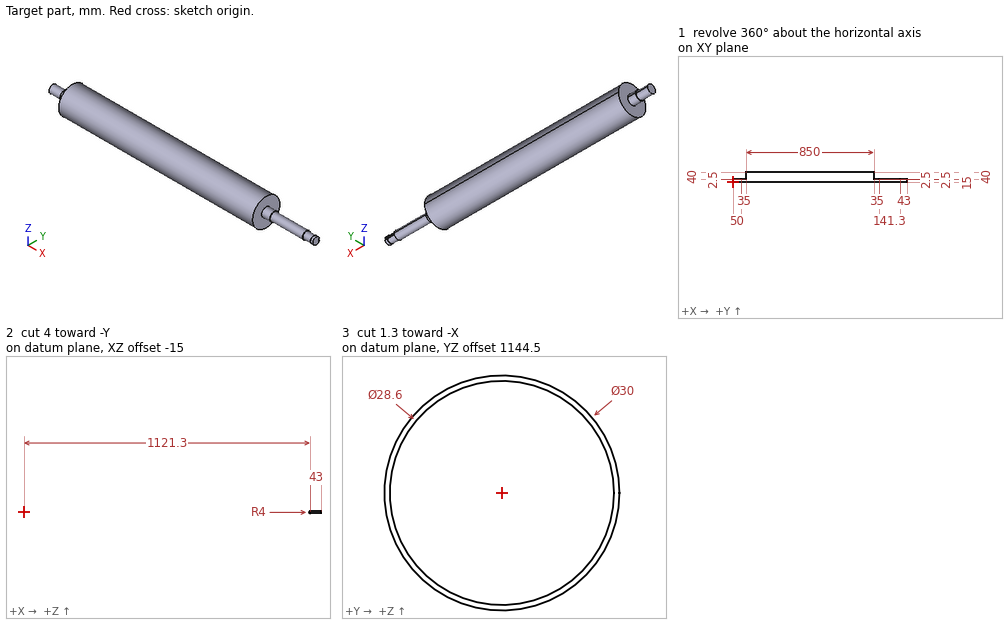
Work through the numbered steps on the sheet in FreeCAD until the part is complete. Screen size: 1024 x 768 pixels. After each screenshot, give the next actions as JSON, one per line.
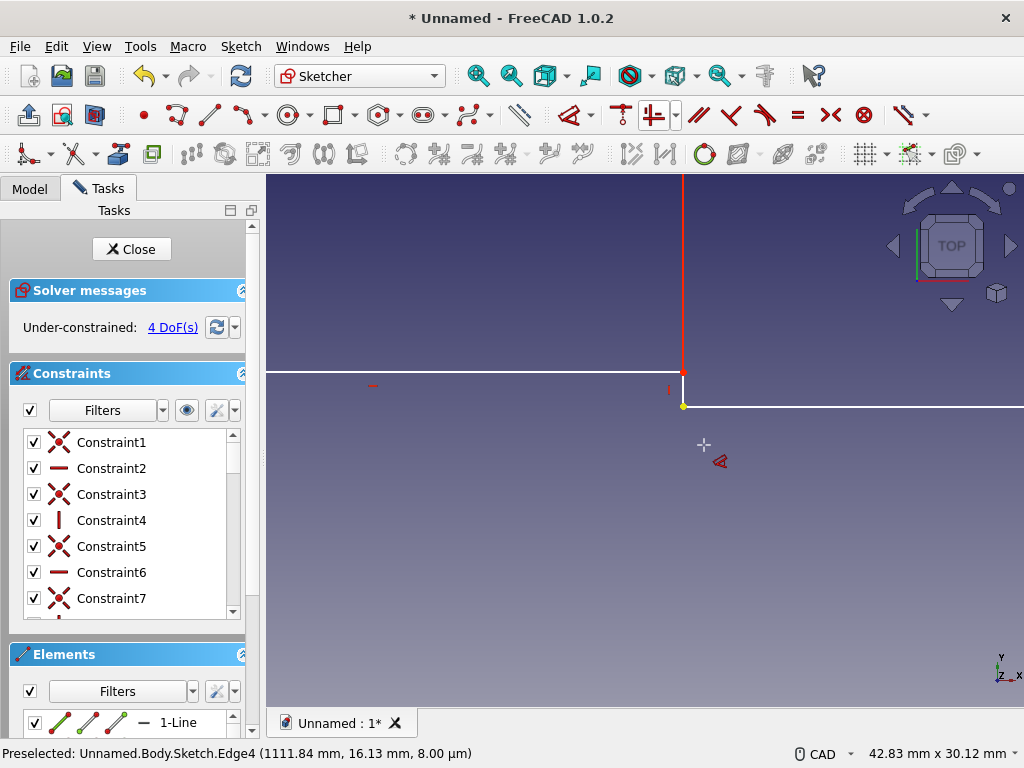
{"action": "left_click", "coordinate": [683, 396]}
{"action": "left_click", "coordinate": [717, 389]}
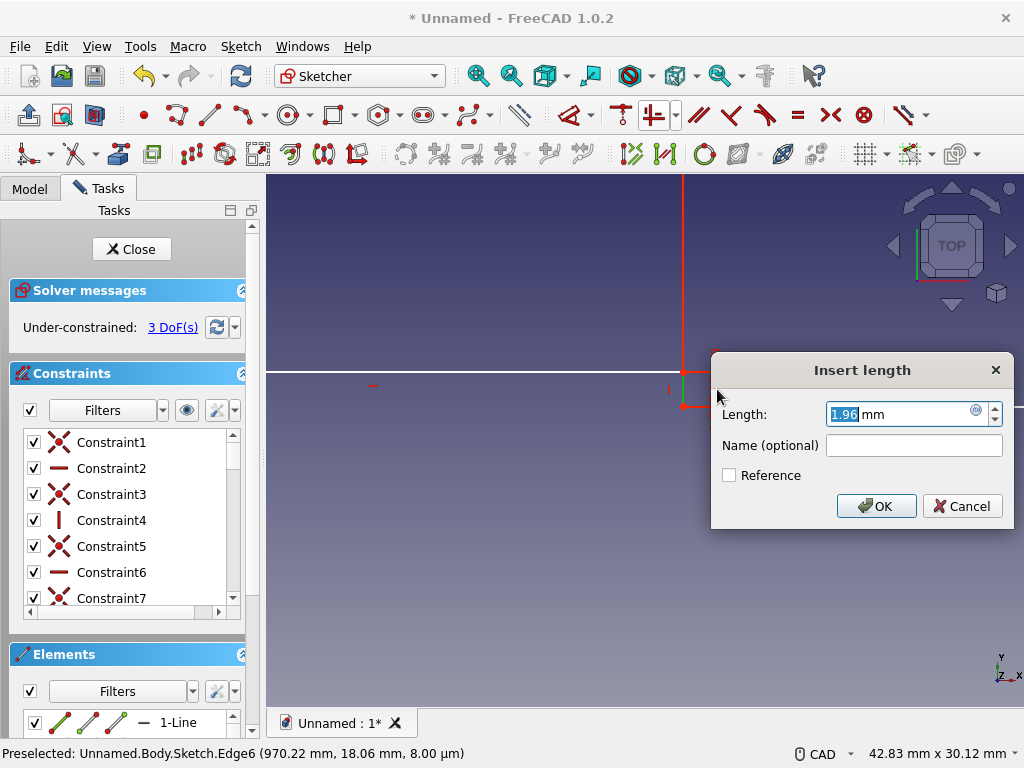
{"action": "type", "text": "2.5"}
{"action": "key", "text": "Return"}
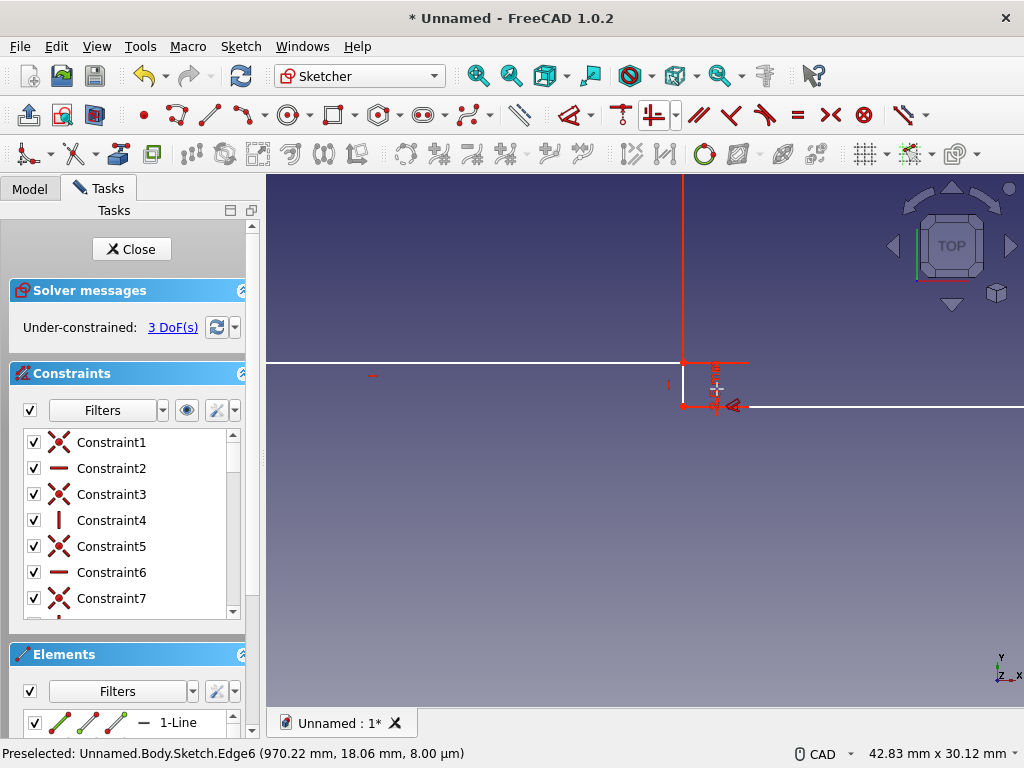
{"action": "scroll", "coordinate": [576, 440], "scroll_direction": "down", "scroll_amount": 15}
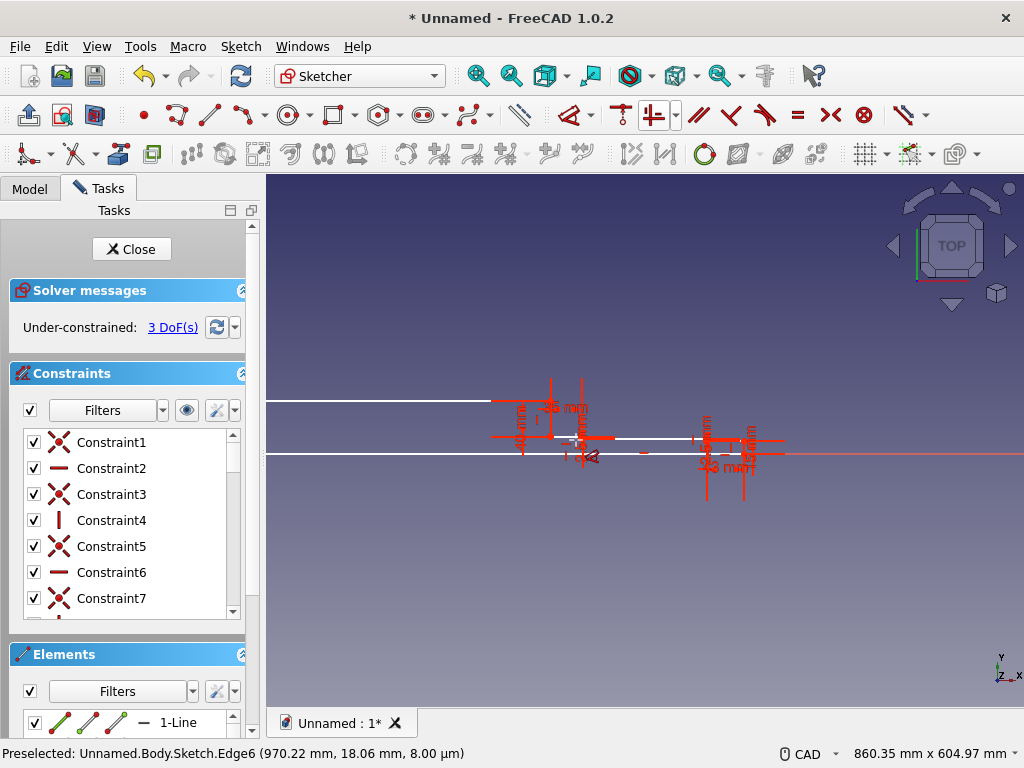
{"action": "scroll", "coordinate": [775, 448], "scroll_direction": "down", "scroll_amount": 5}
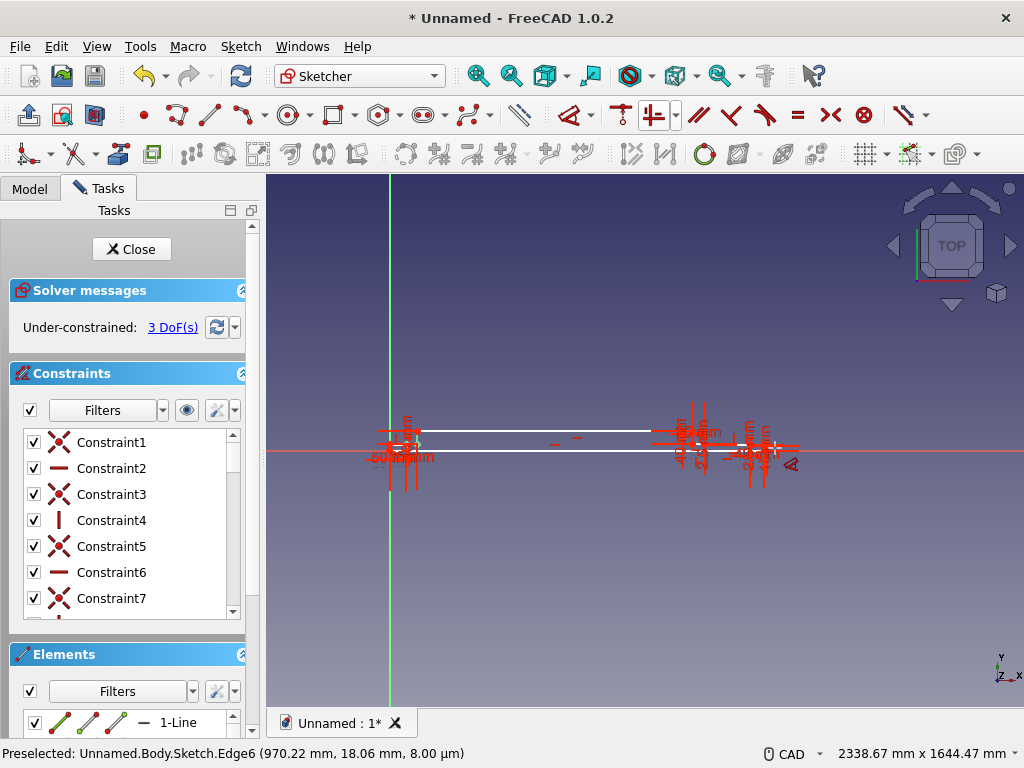
{"action": "left_click", "coordinate": [610, 431]}
{"action": "left_click", "coordinate": [555, 397]}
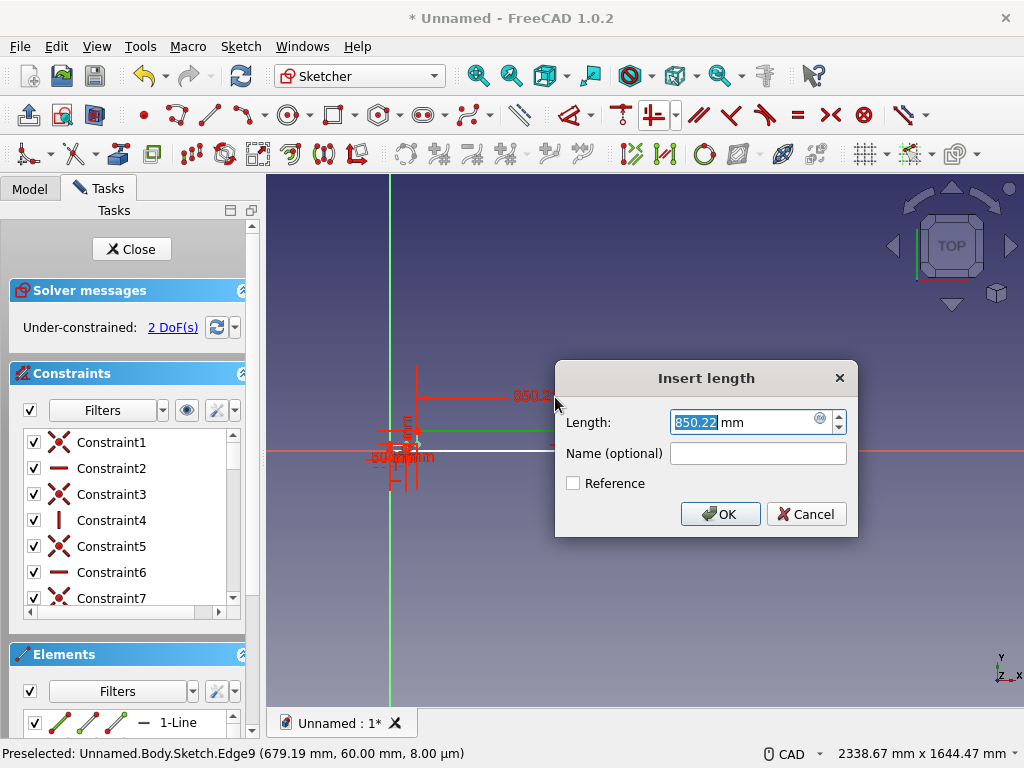
{"action": "type", "text": "850"}
{"action": "key", "text": "Return"}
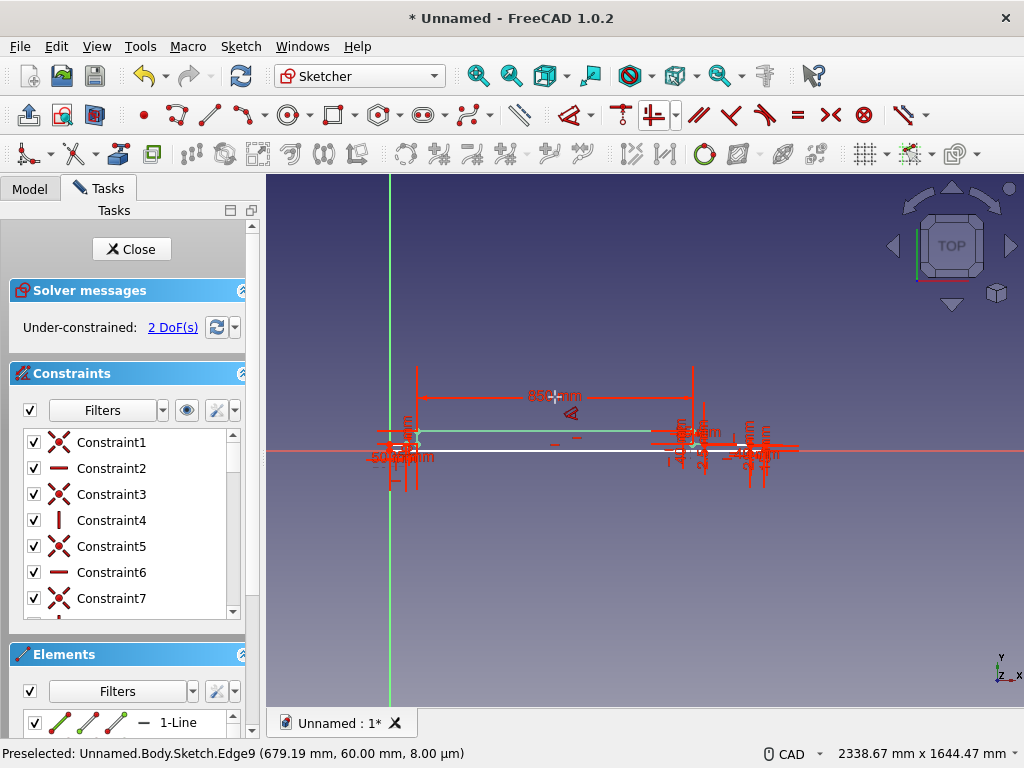
{"action": "scroll", "coordinate": [406, 445], "scroll_direction": "up", "scroll_amount": 20}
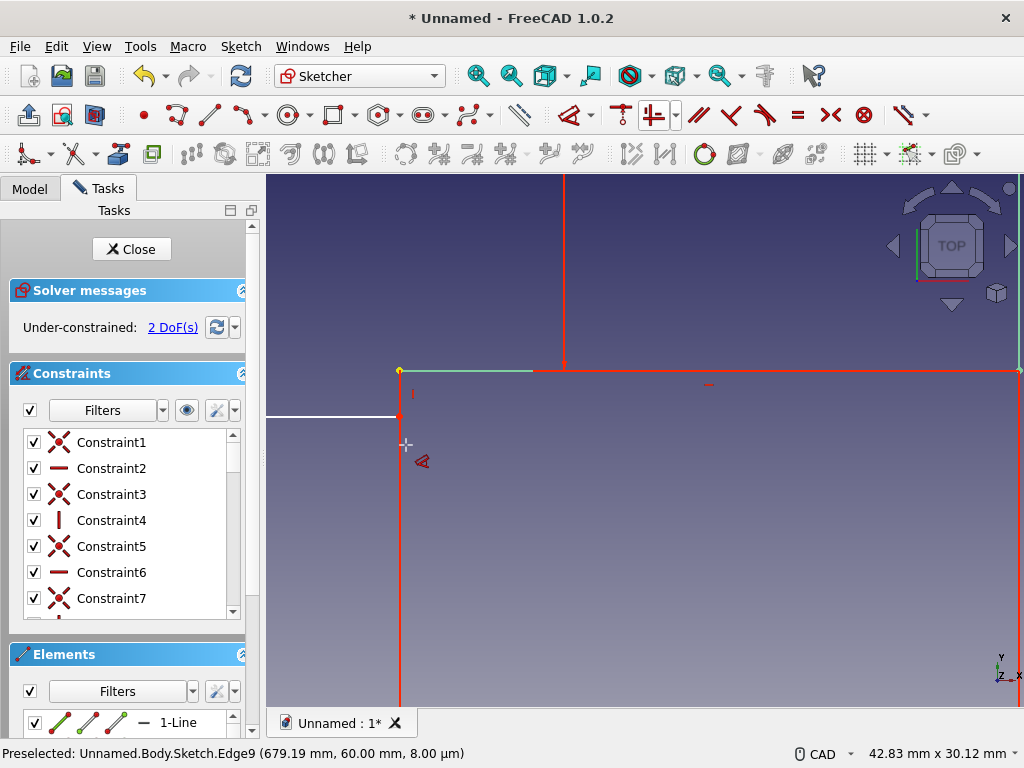
{"action": "left_click", "coordinate": [400, 394]}
{"action": "left_click", "coordinate": [366, 394]}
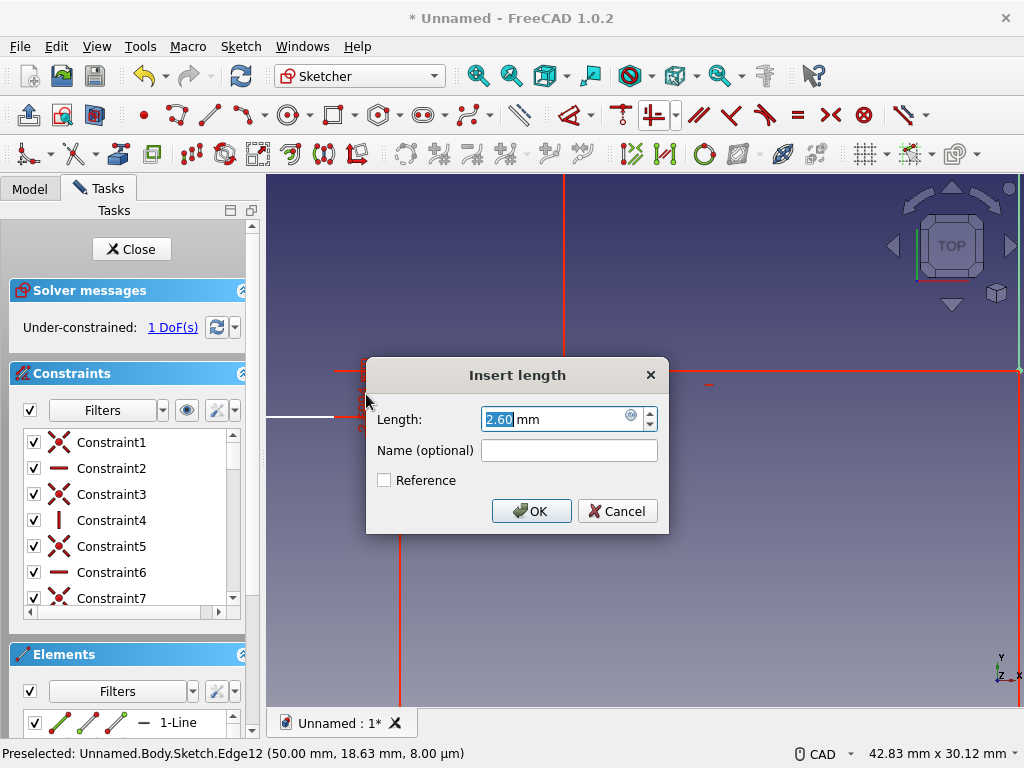
{"action": "type", "text": "2.5"}
{"action": "key", "text": "Return"}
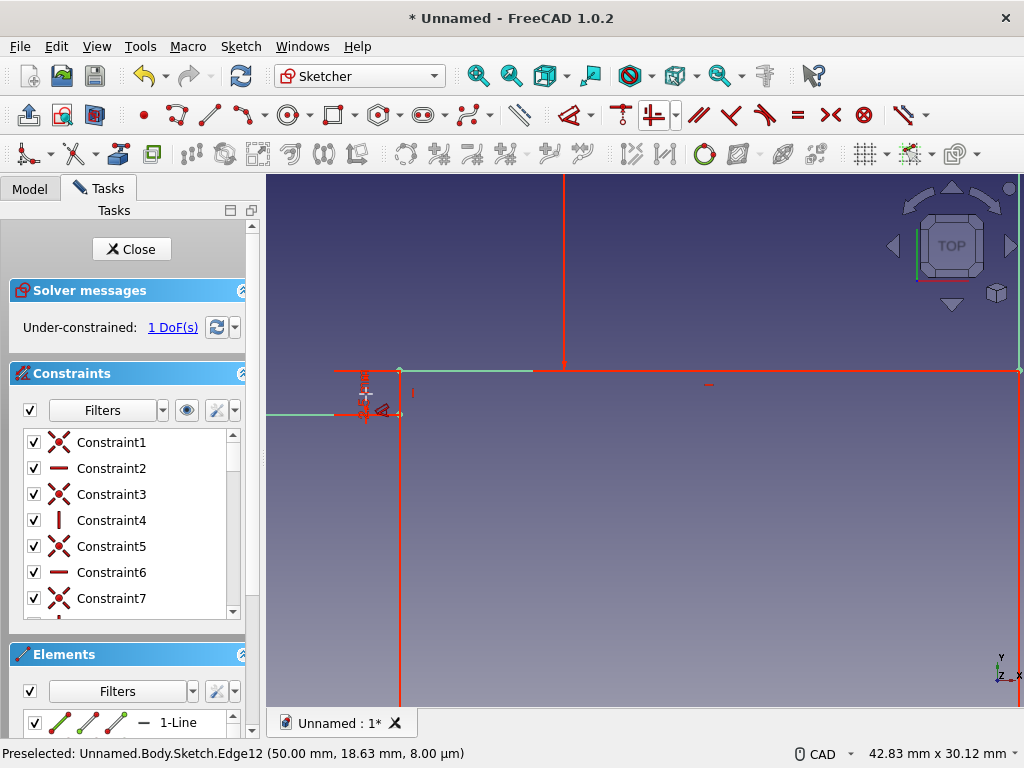
{"action": "scroll", "coordinate": [576, 440], "scroll_direction": "down", "scroll_amount": 15}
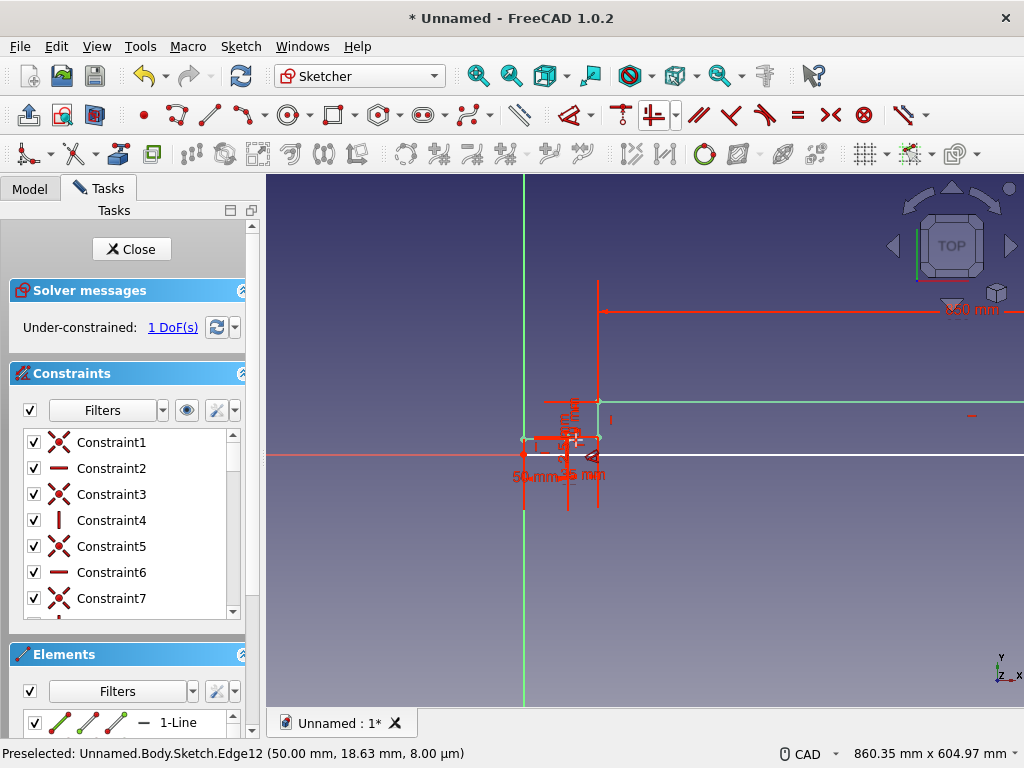
{"action": "scroll", "coordinate": [311, 448], "scroll_direction": "down", "scroll_amount": 5}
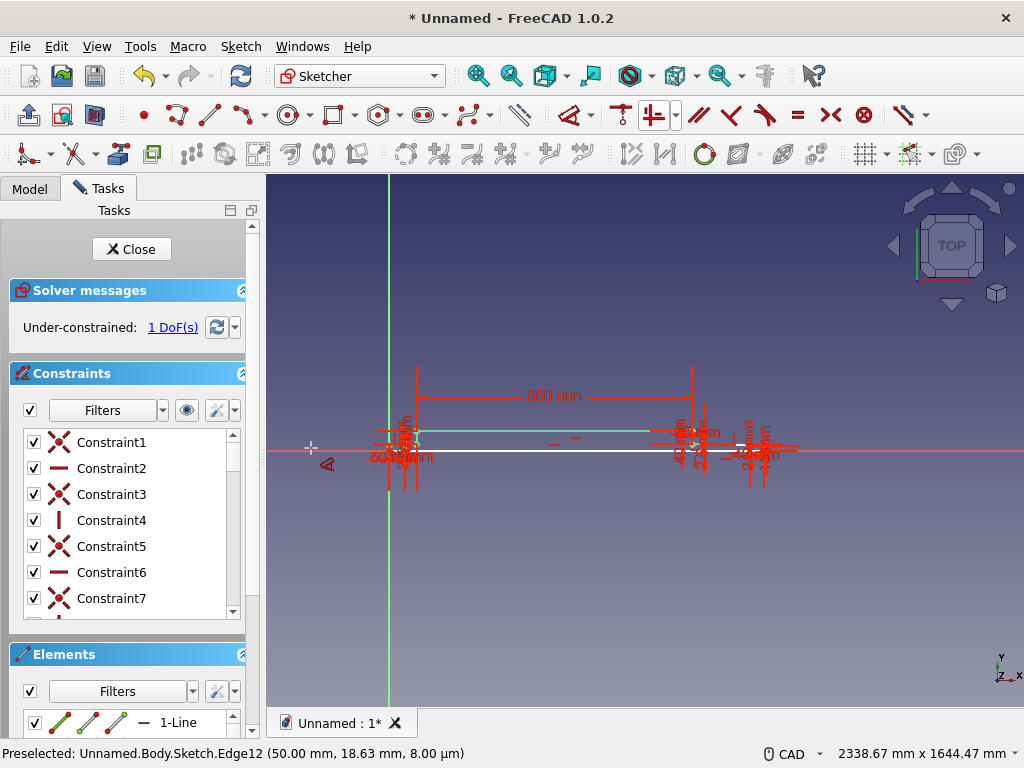
{"action": "scroll", "coordinate": [736, 445], "scroll_direction": "up", "scroll_amount": 5}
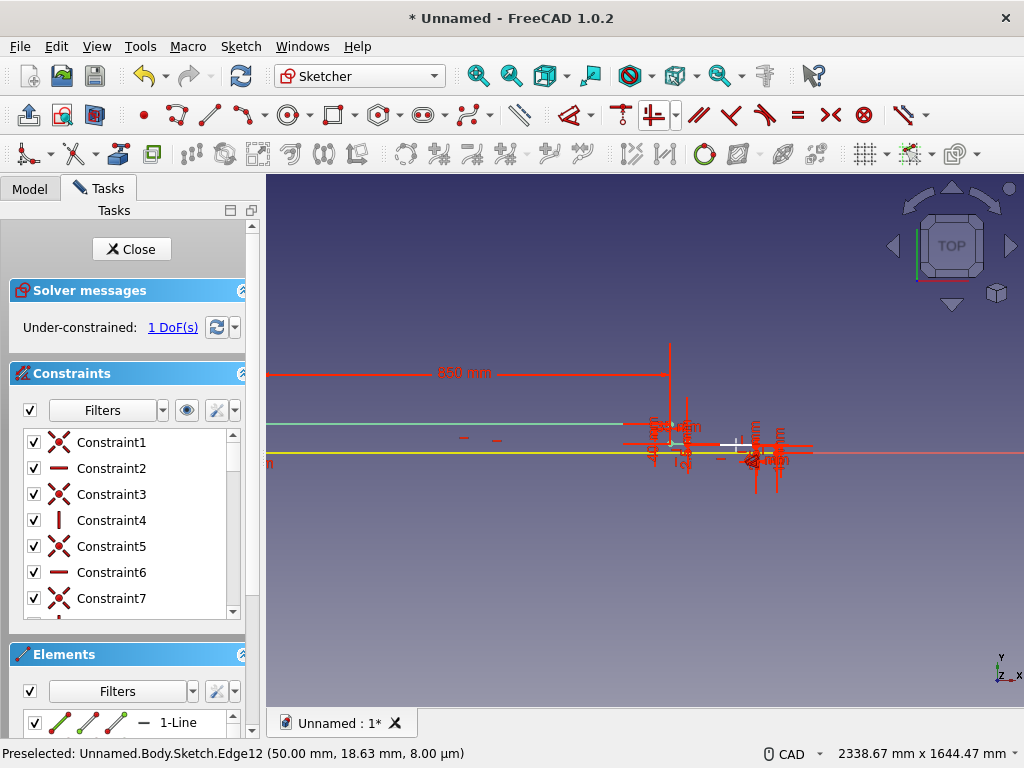
{"action": "left_click", "coordinate": [734, 444]}
{"action": "left_click", "coordinate": [709, 478]}